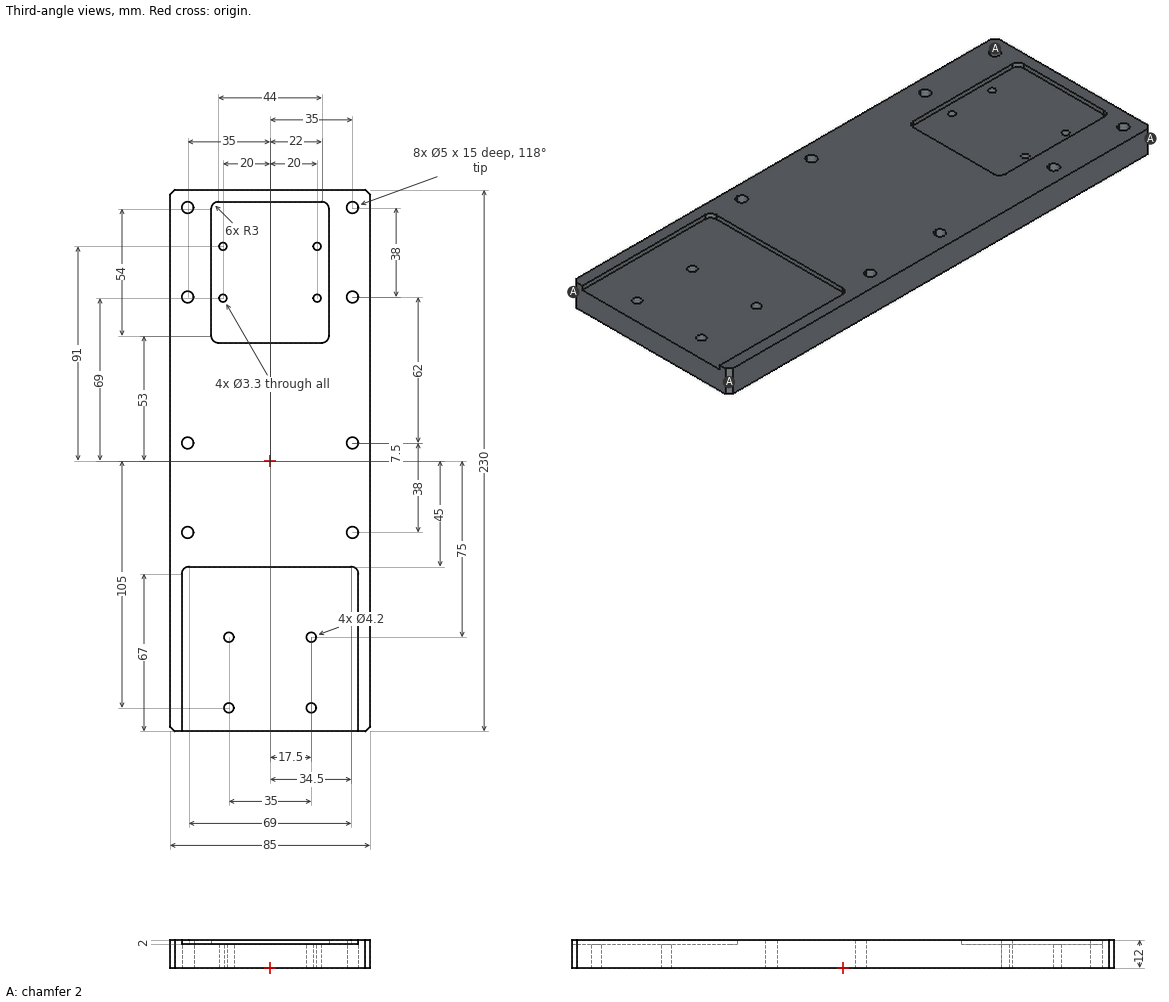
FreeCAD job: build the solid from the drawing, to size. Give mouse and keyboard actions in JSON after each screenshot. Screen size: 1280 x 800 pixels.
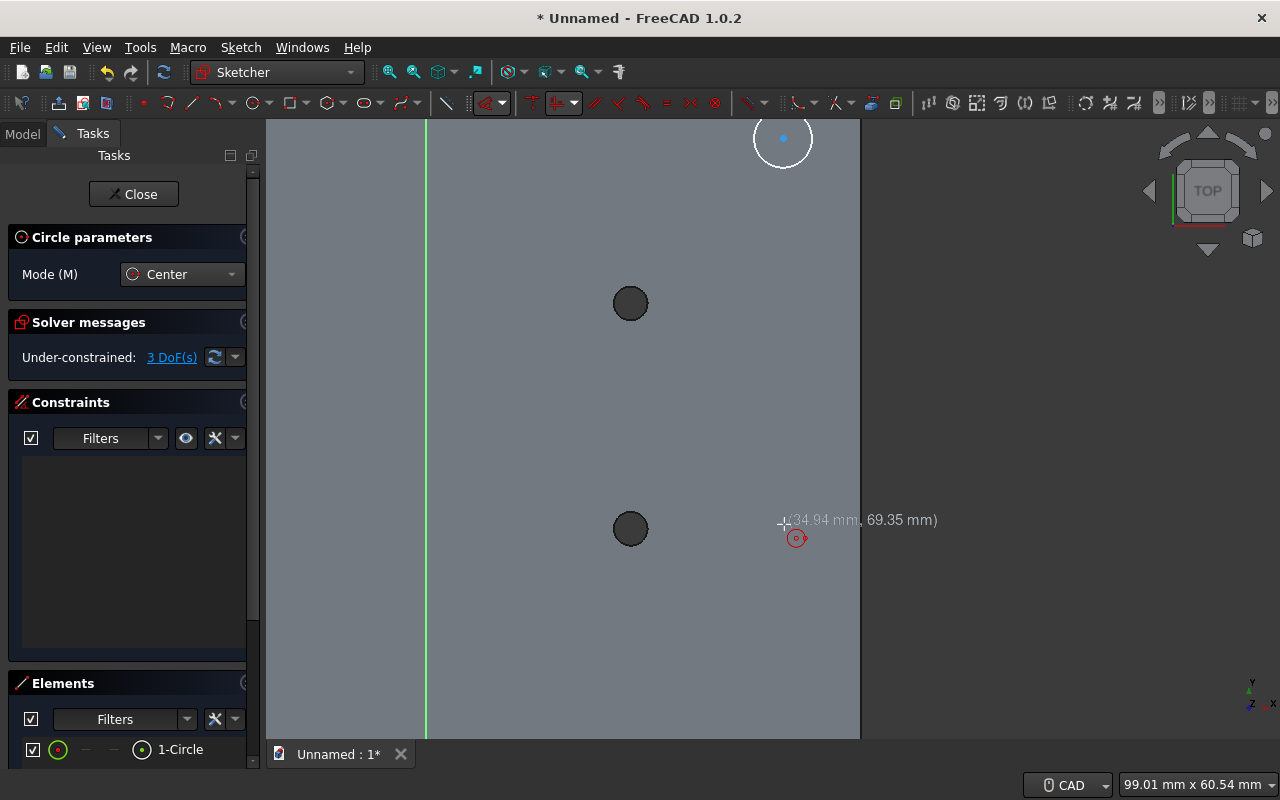
{"action": "scroll", "coordinate": [796, 294], "scroll_direction": "down", "scroll_amount": 7}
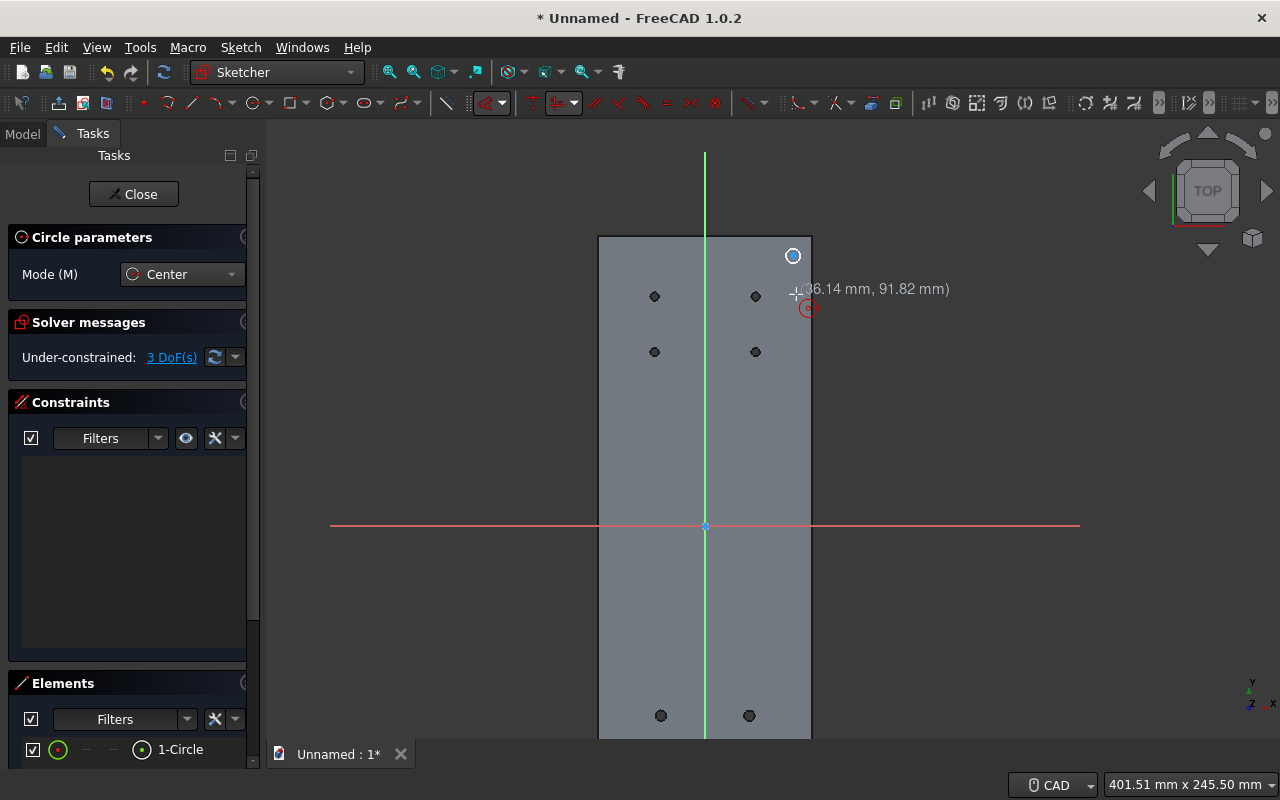
{"action": "left_click", "coordinate": [794, 351]}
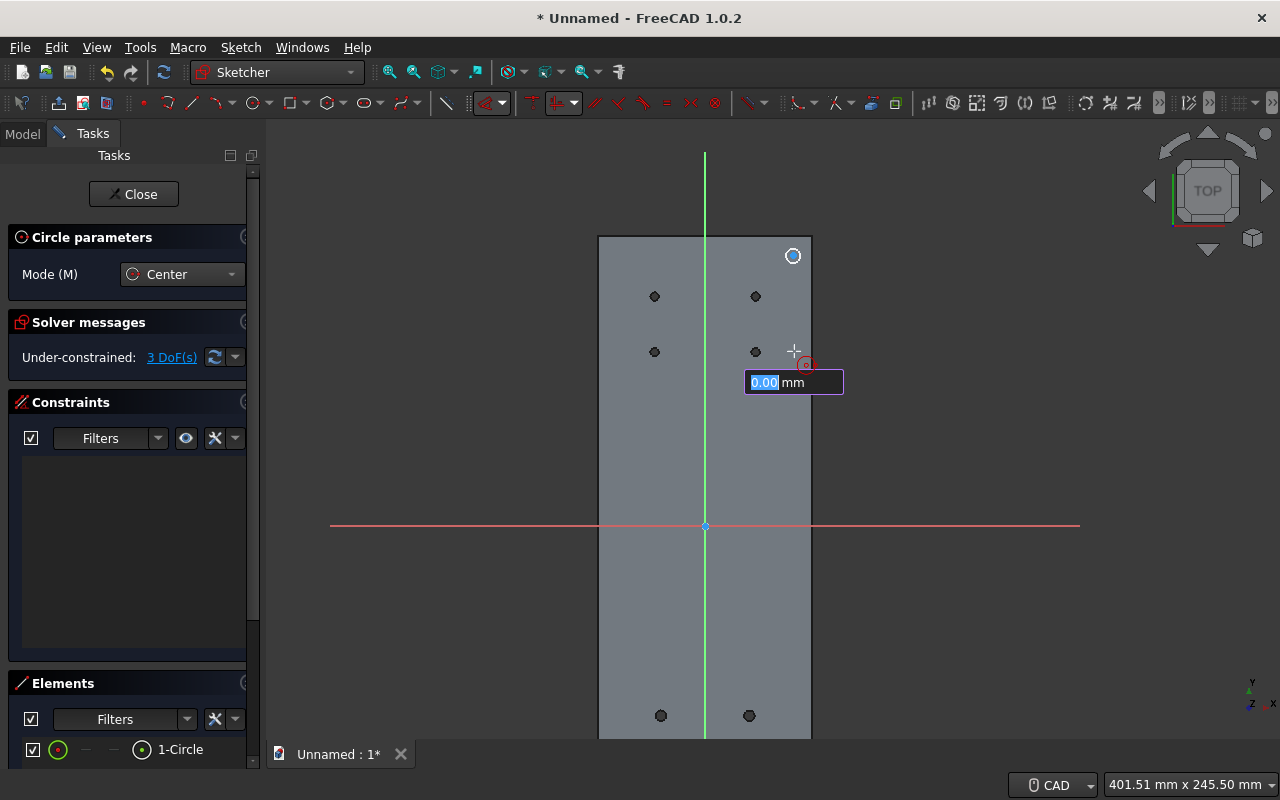
{"action": "scroll", "coordinate": [798, 346], "scroll_direction": "up", "scroll_amount": 5}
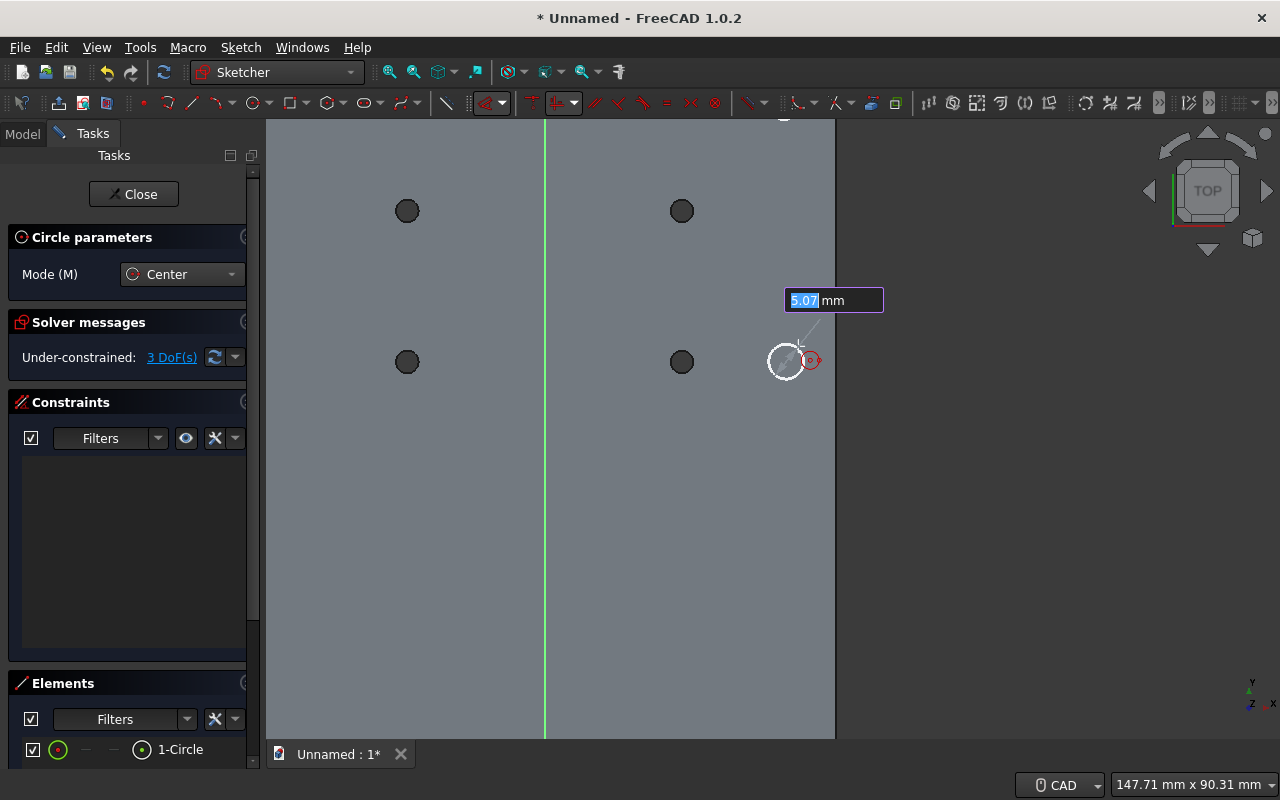
{"action": "left_click", "coordinate": [797, 346]}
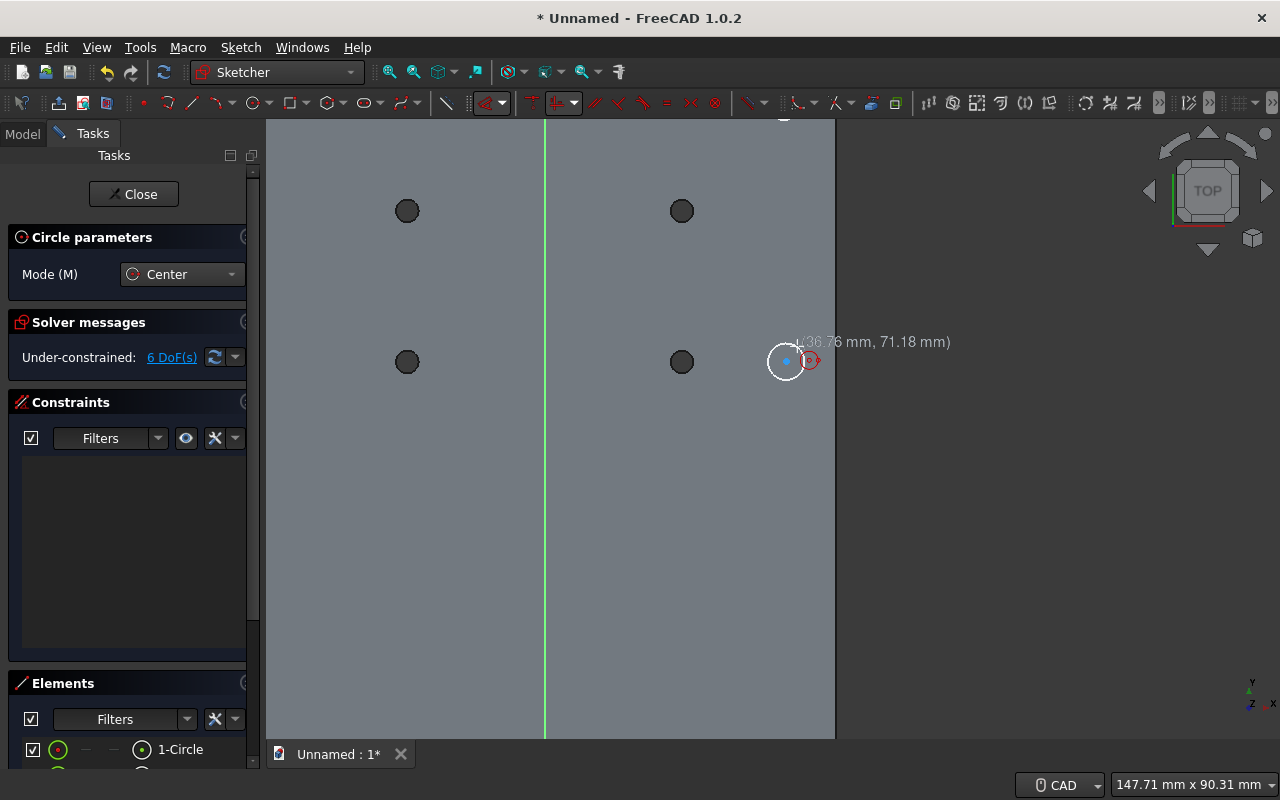
{"action": "scroll", "coordinate": [304, 359], "scroll_direction": "up", "scroll_amount": 2}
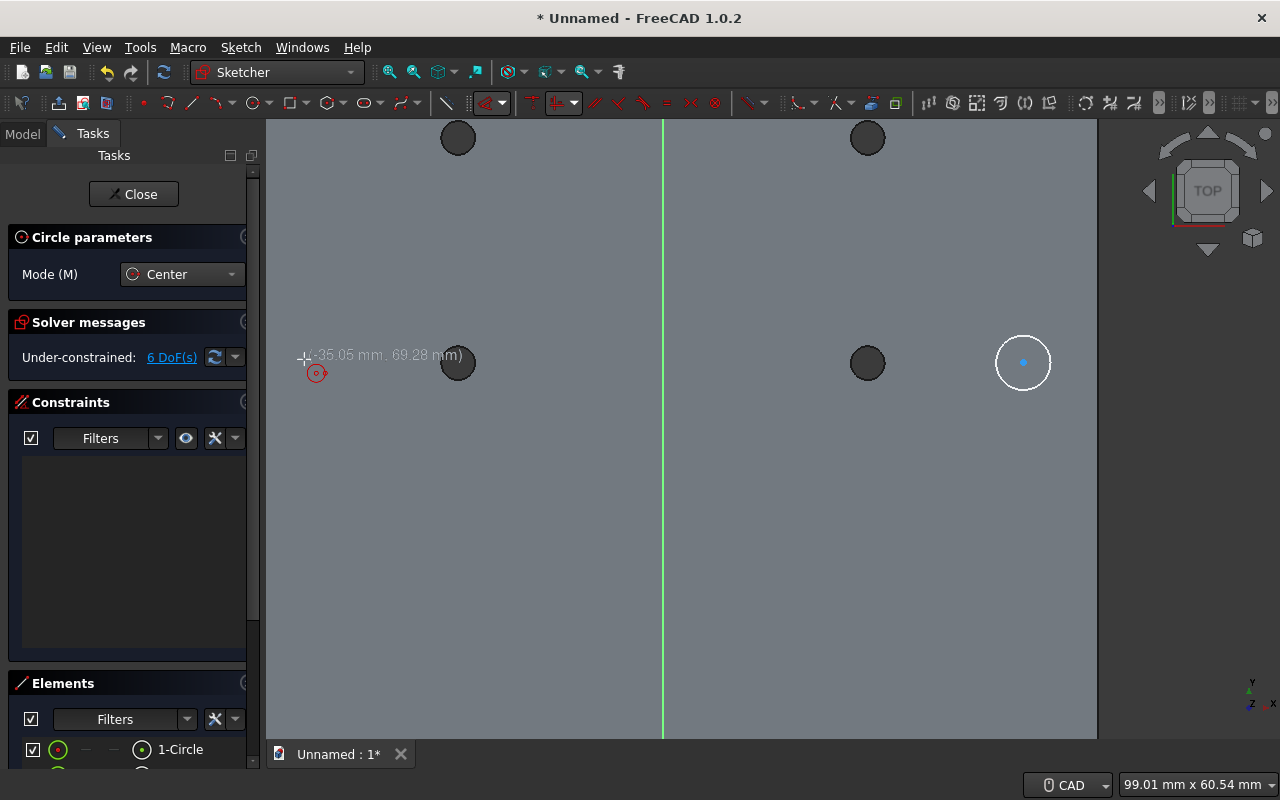
{"action": "scroll", "coordinate": [718, 348], "scroll_direction": "down", "scroll_amount": 7}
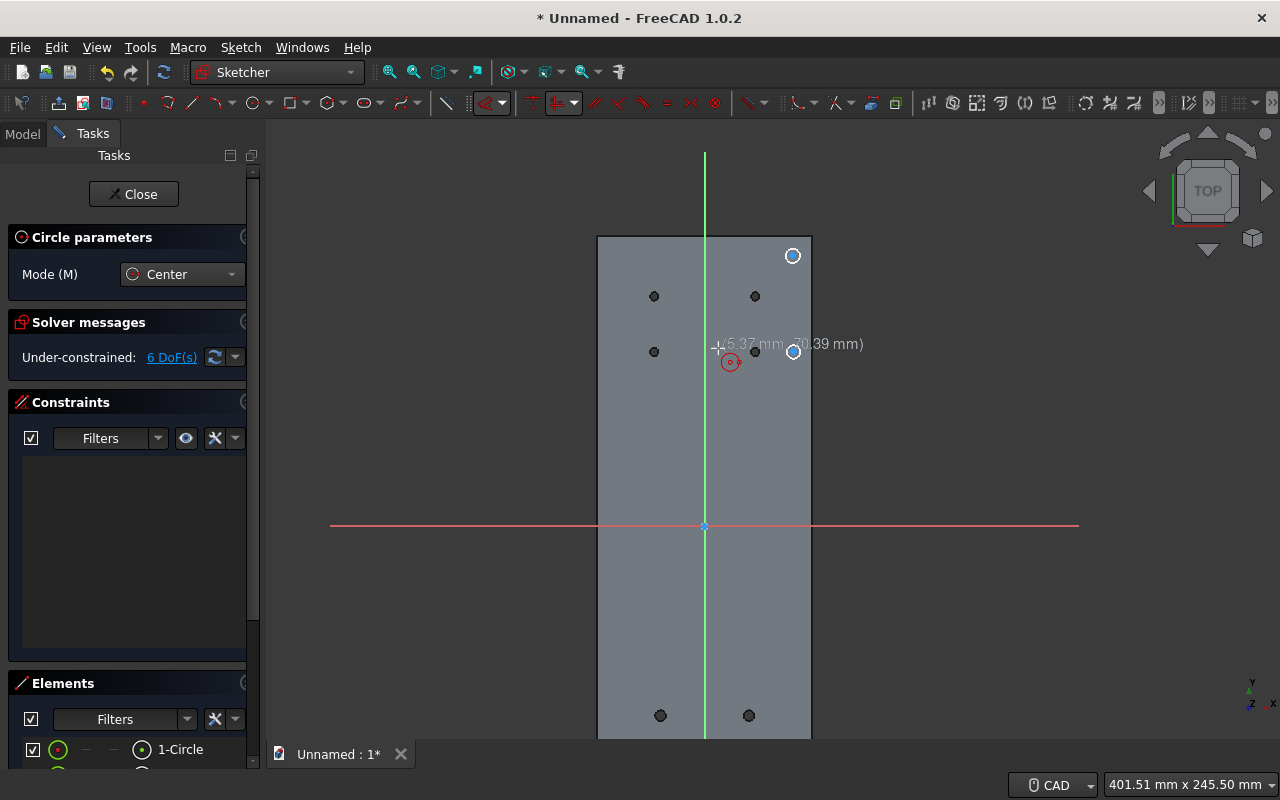
{"action": "left_click", "coordinate": [616, 351]}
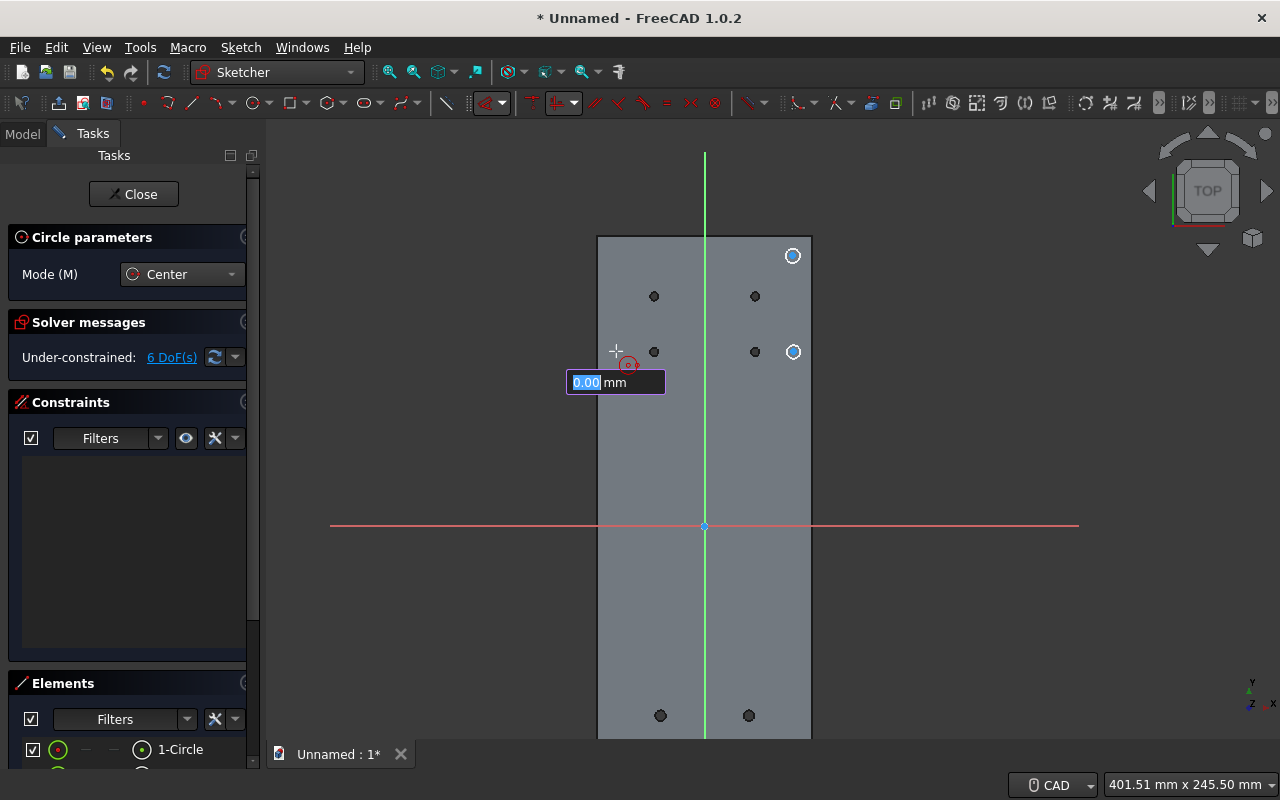
{"action": "scroll", "coordinate": [621, 346], "scroll_direction": "up", "scroll_amount": 5}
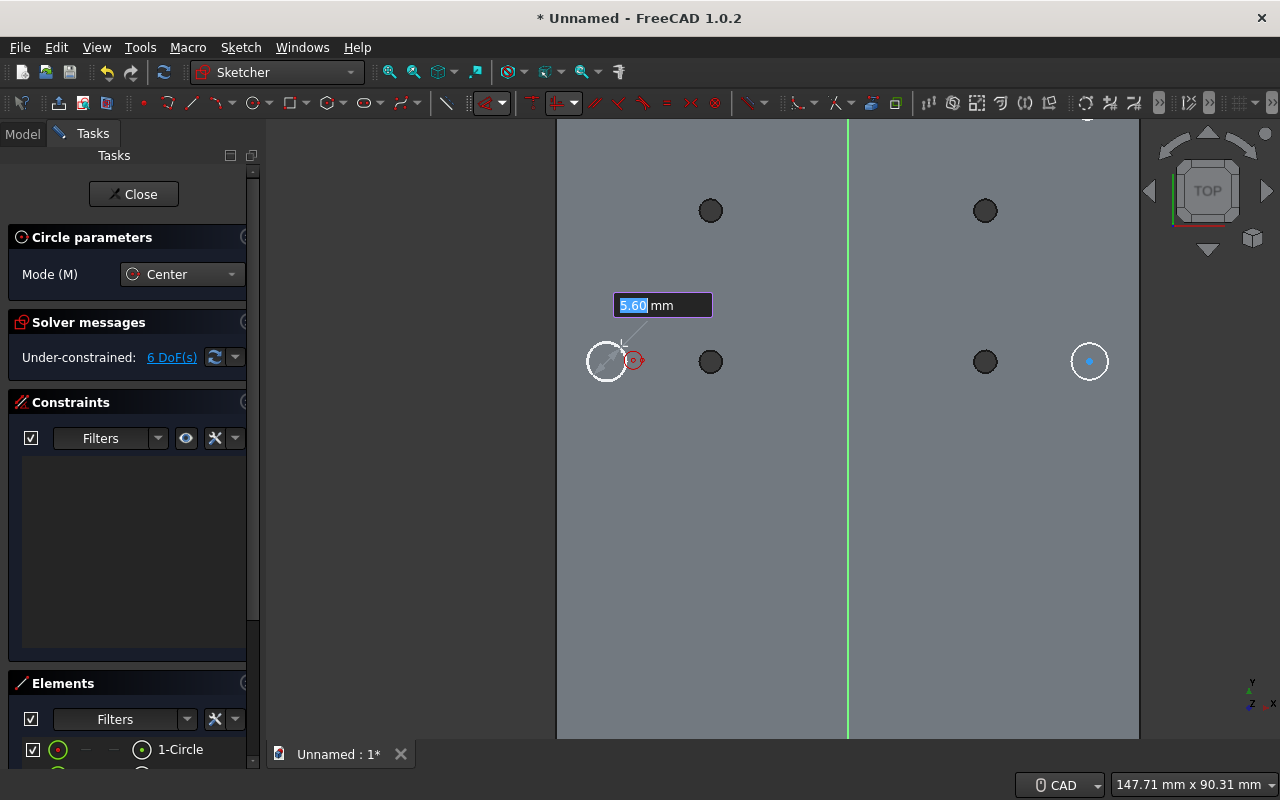
{"action": "left_click", "coordinate": [620, 346]}